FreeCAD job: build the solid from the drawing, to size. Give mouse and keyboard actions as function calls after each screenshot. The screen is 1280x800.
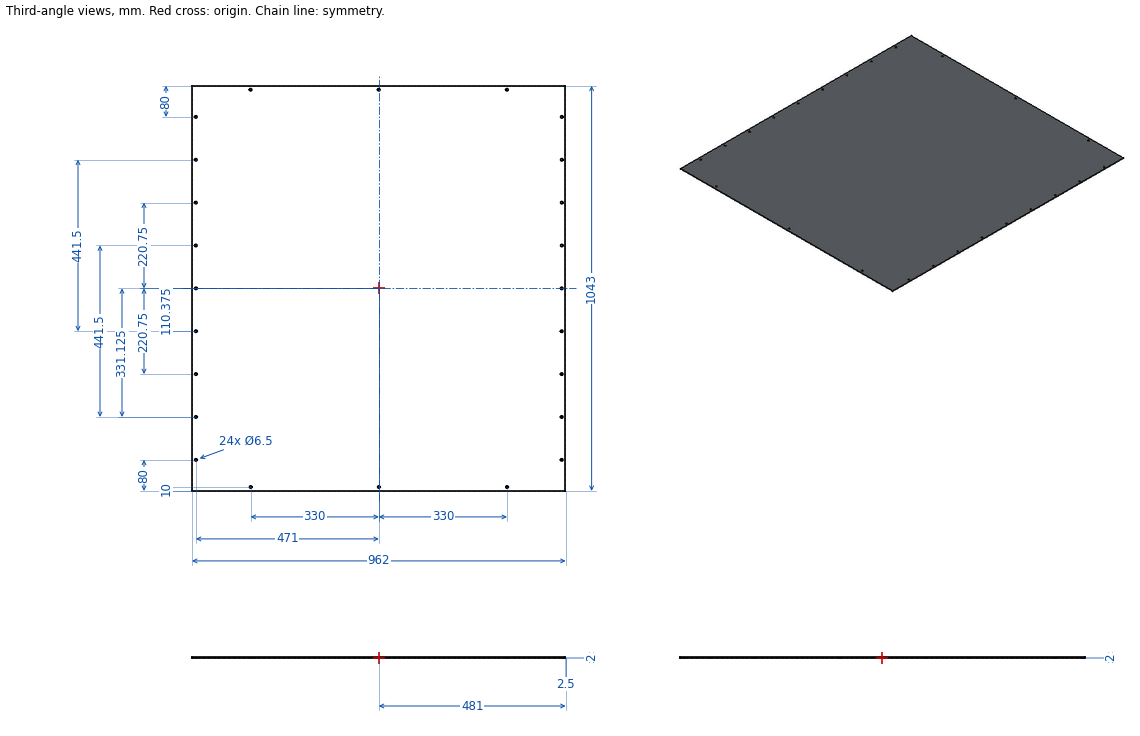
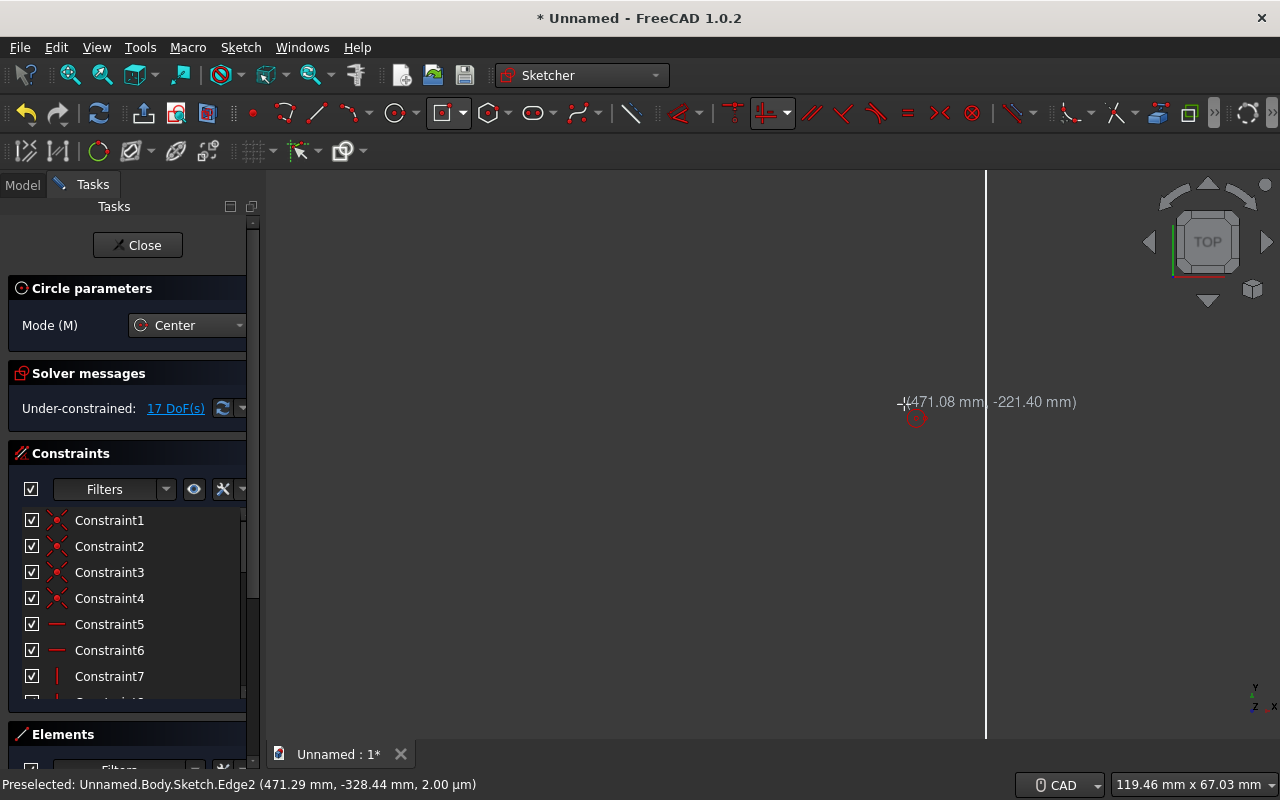
scroll(904, 555, down, 15)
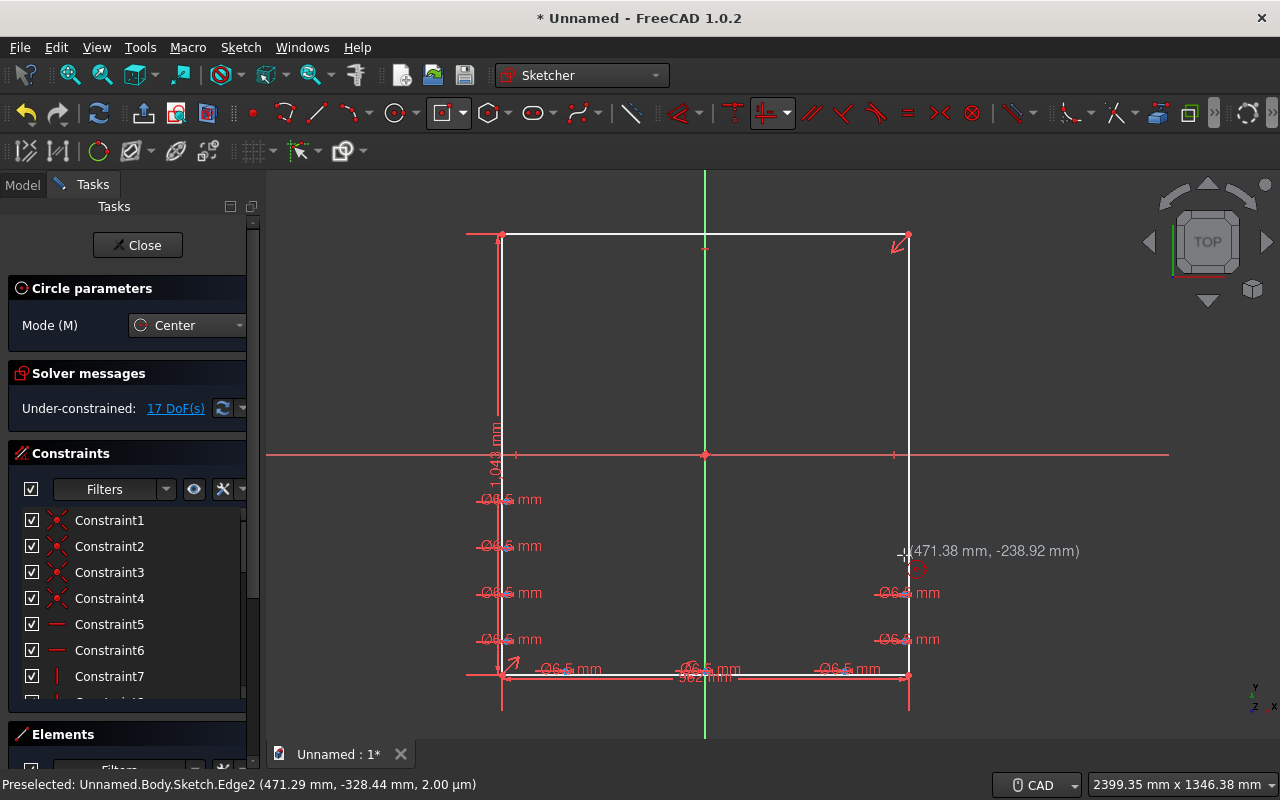
scroll(904, 548, up, 7)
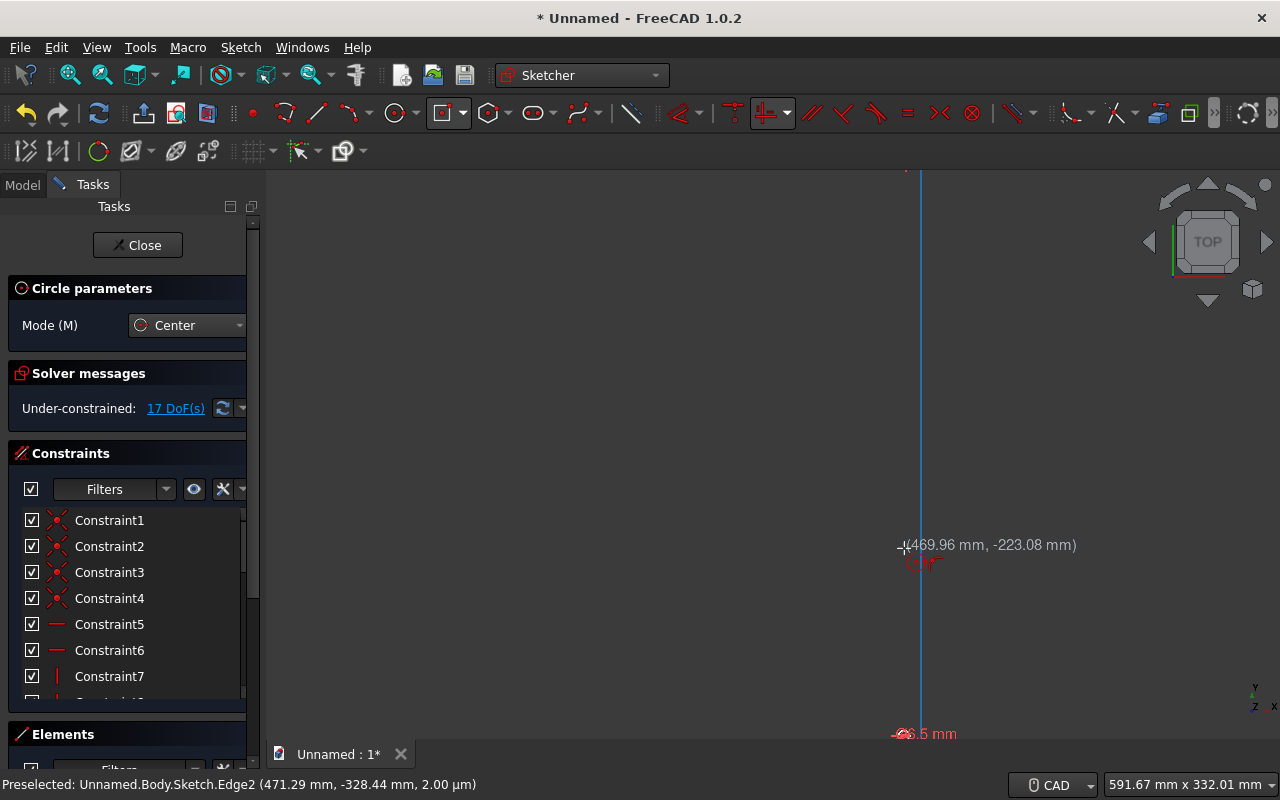
click(904, 546)
move(900, 542)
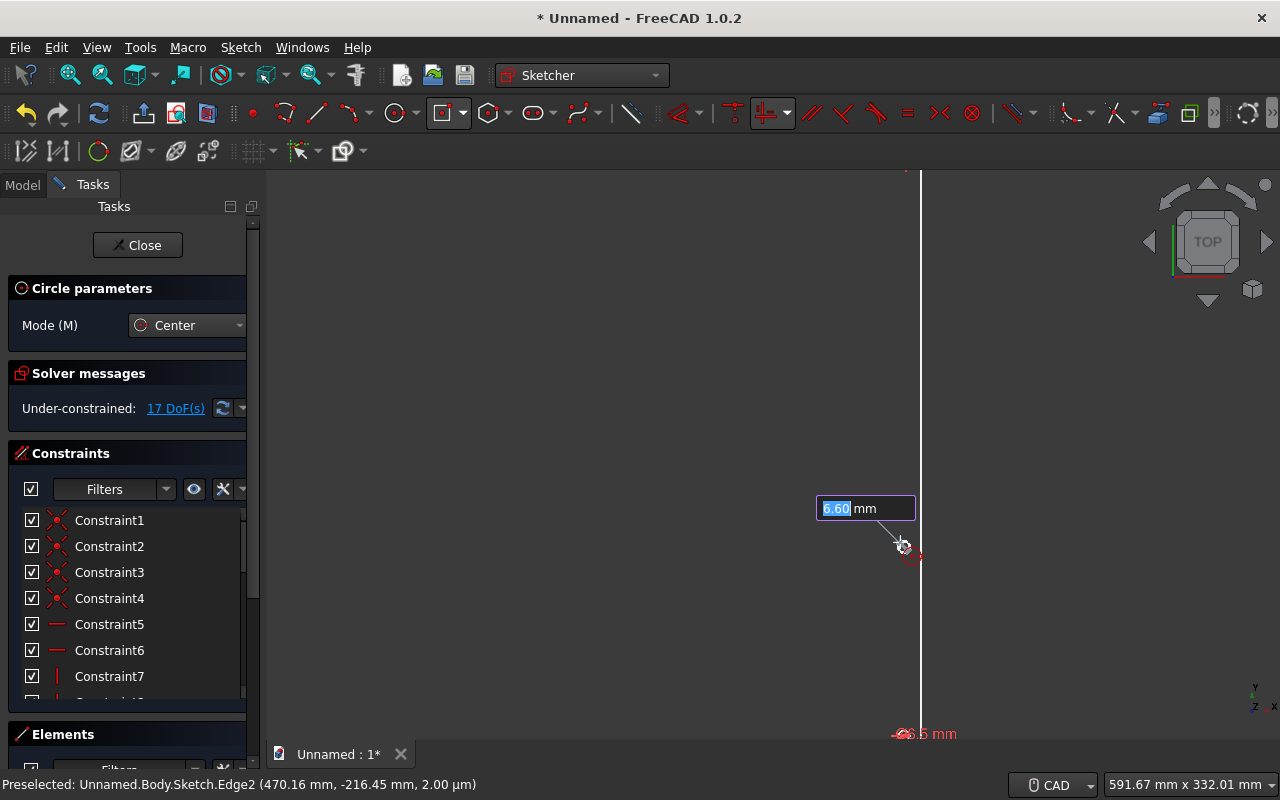
text(6.5)
key(Return)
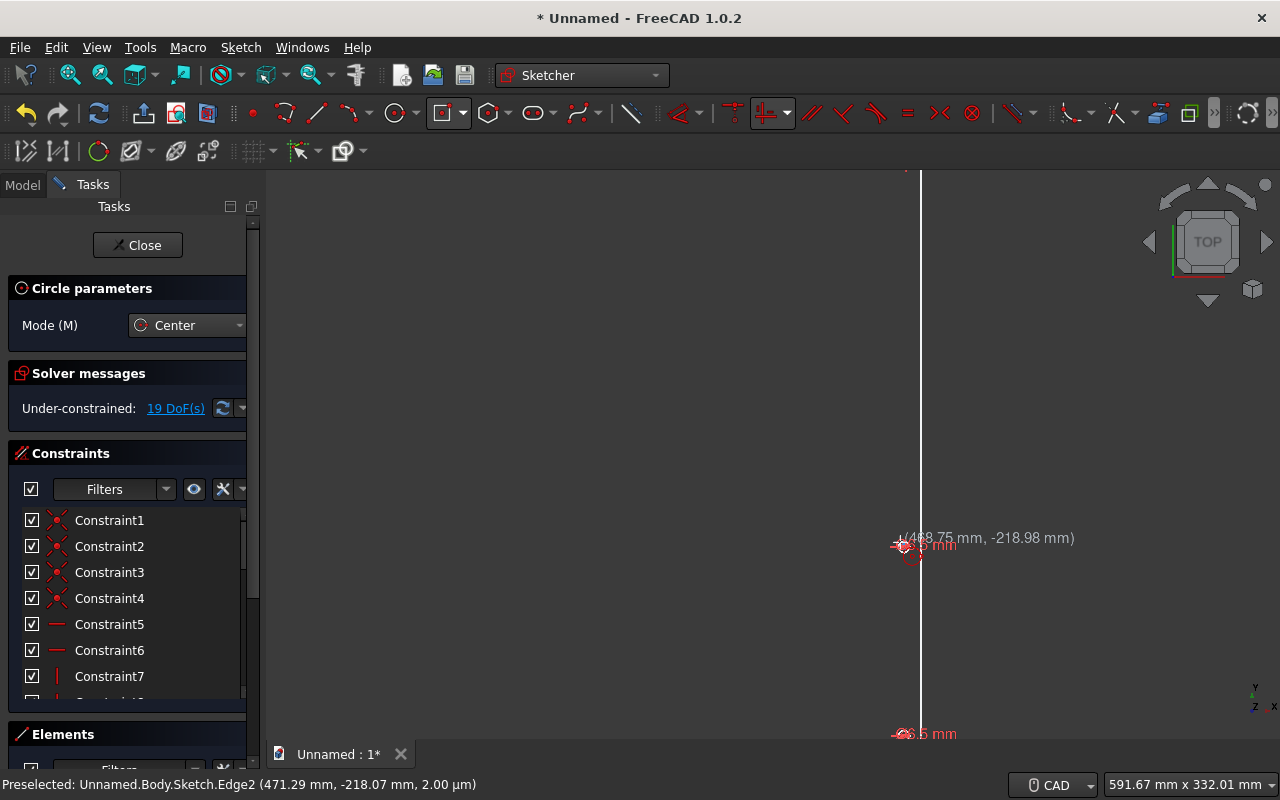
scroll(904, 357, up, 8)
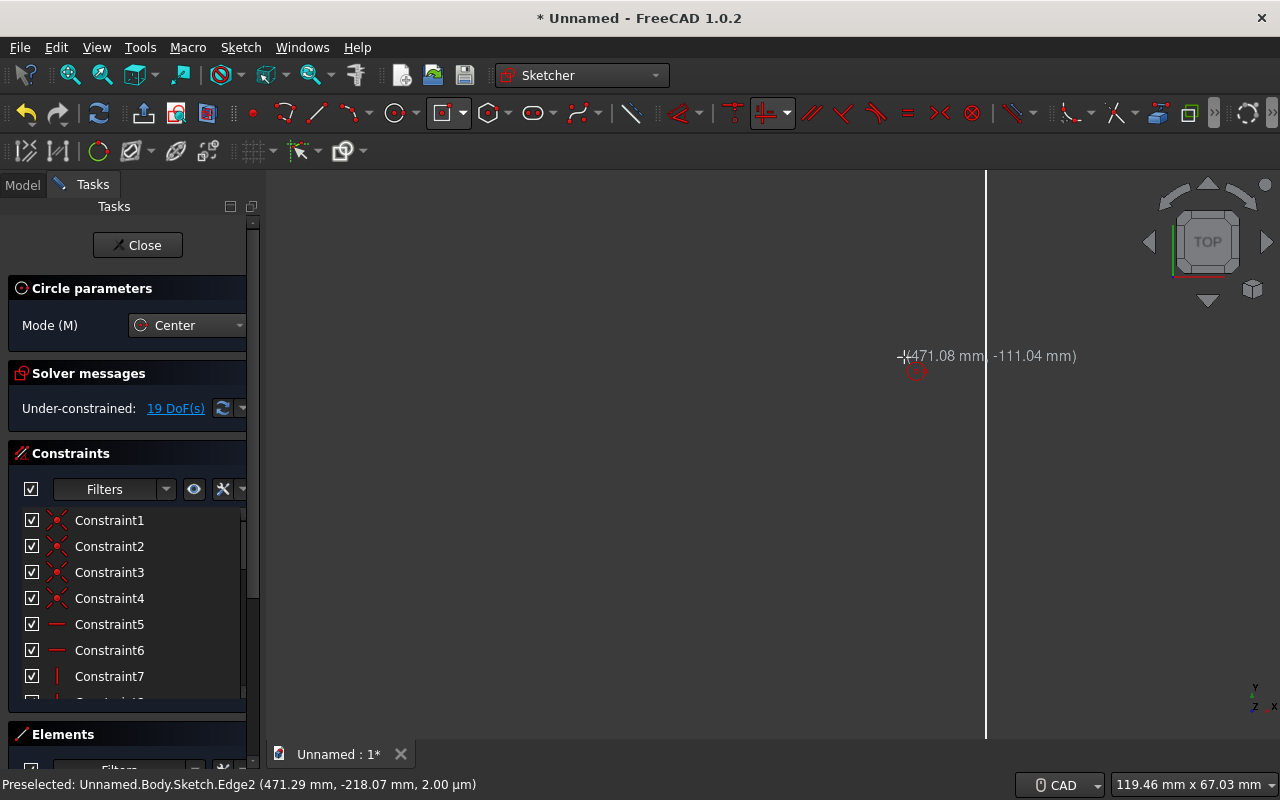
scroll(904, 509, down, 15)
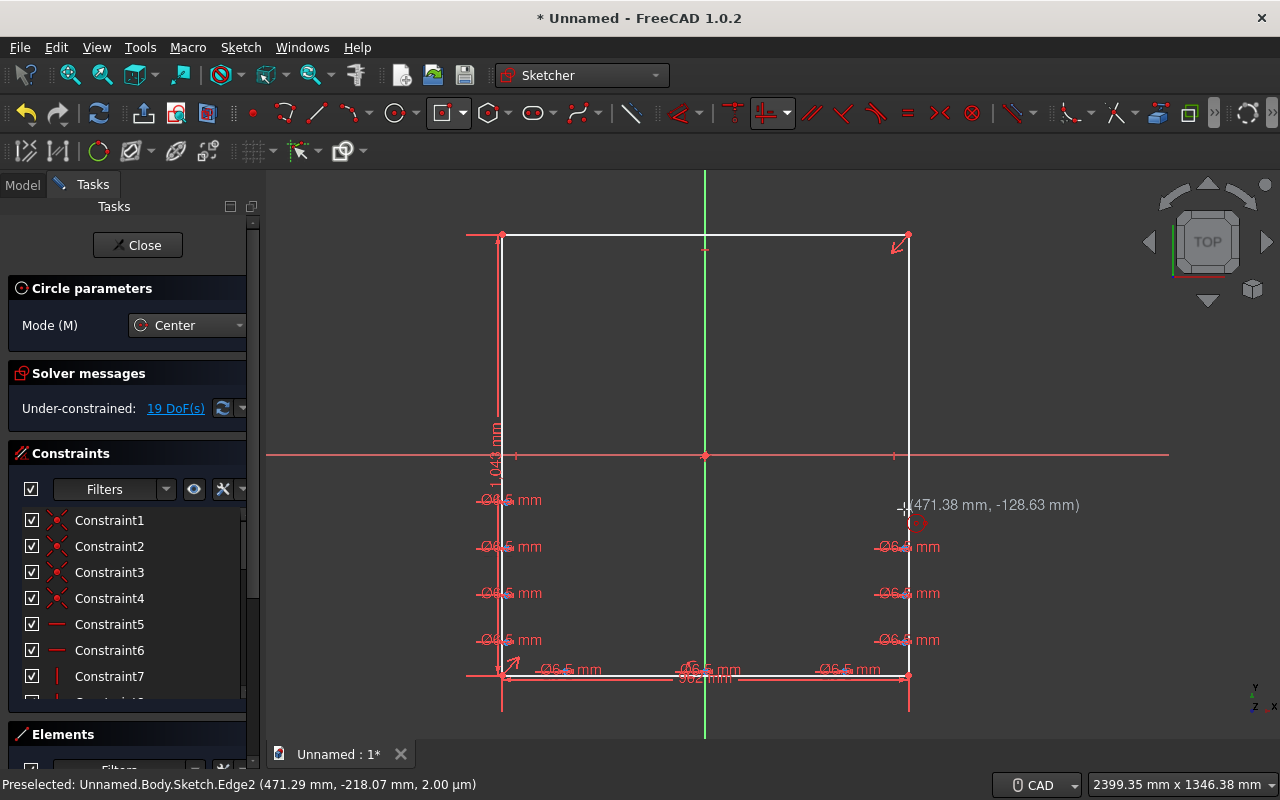
scroll(904, 502, up, 7)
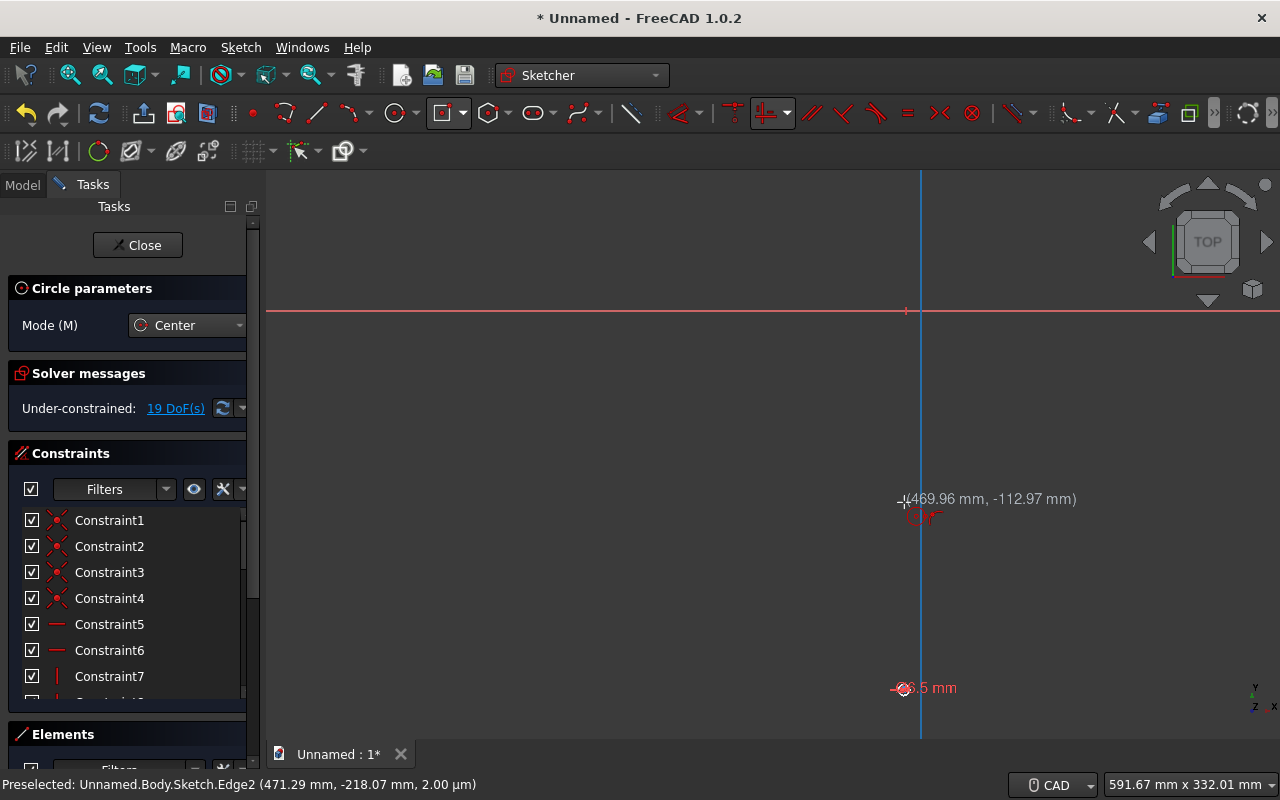
click(904, 500)
move(900, 496)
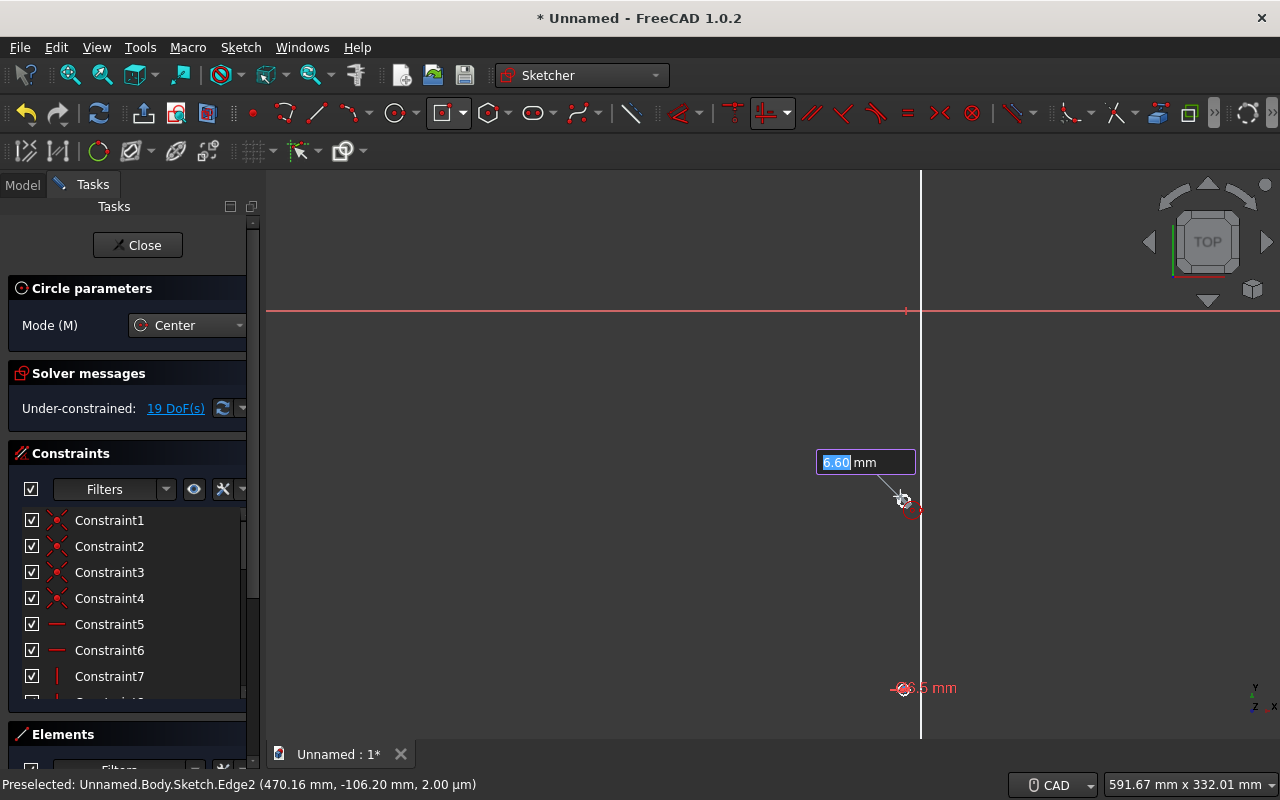
text(6.5)
key(Return)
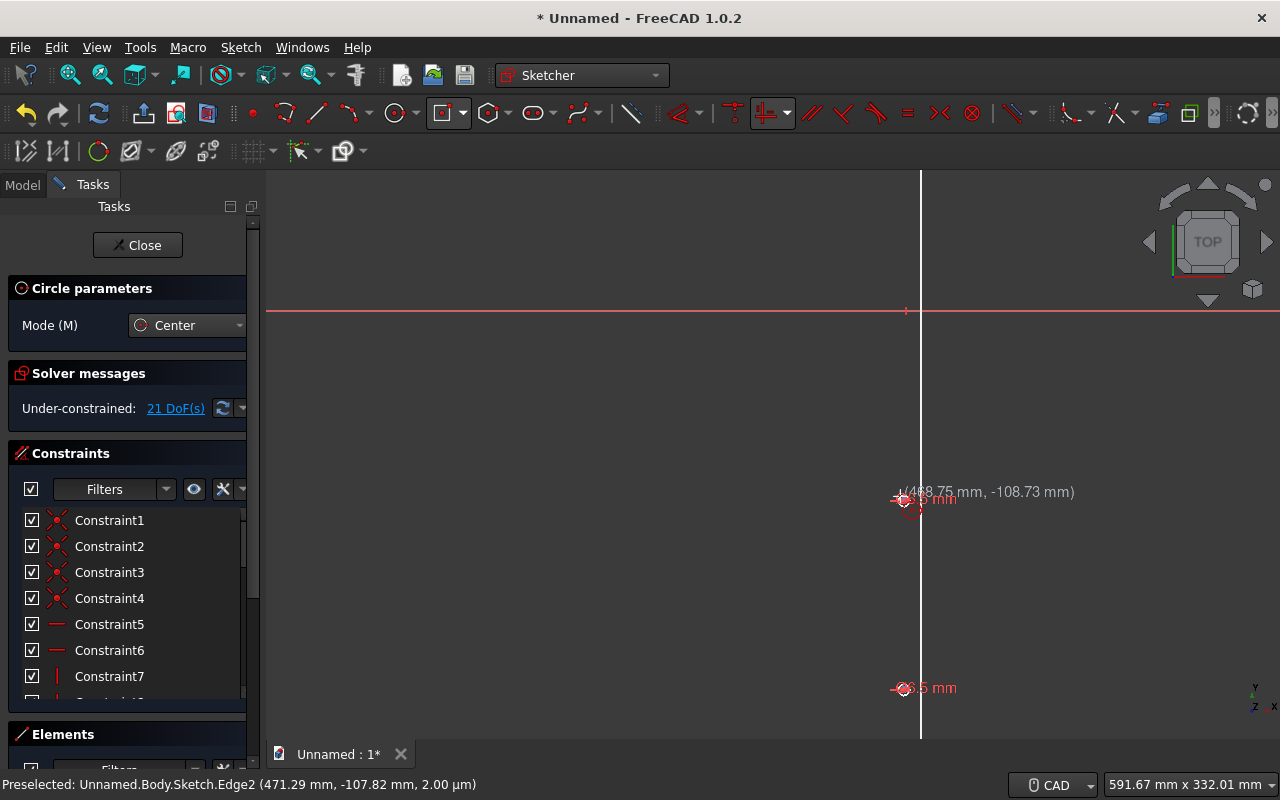
scroll(858, 491, down, 8)